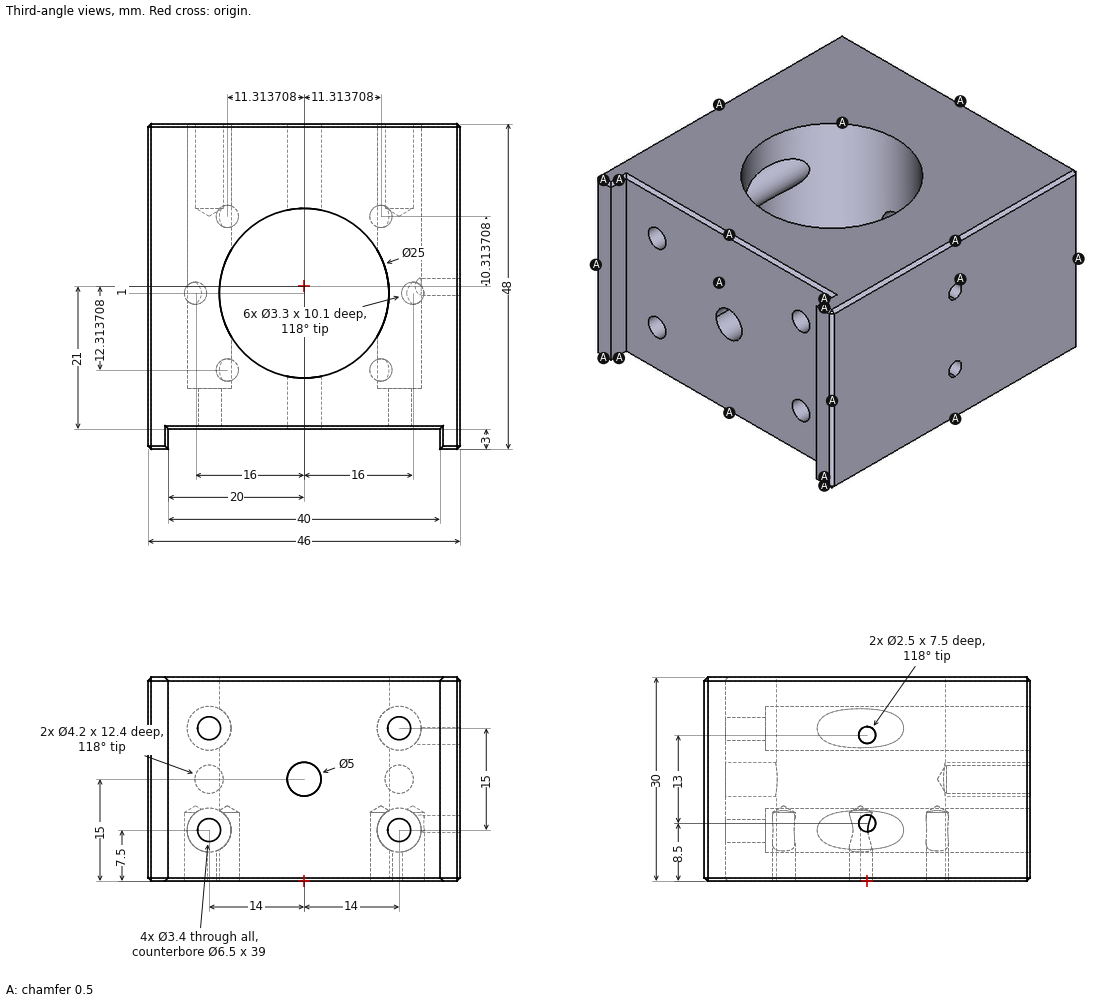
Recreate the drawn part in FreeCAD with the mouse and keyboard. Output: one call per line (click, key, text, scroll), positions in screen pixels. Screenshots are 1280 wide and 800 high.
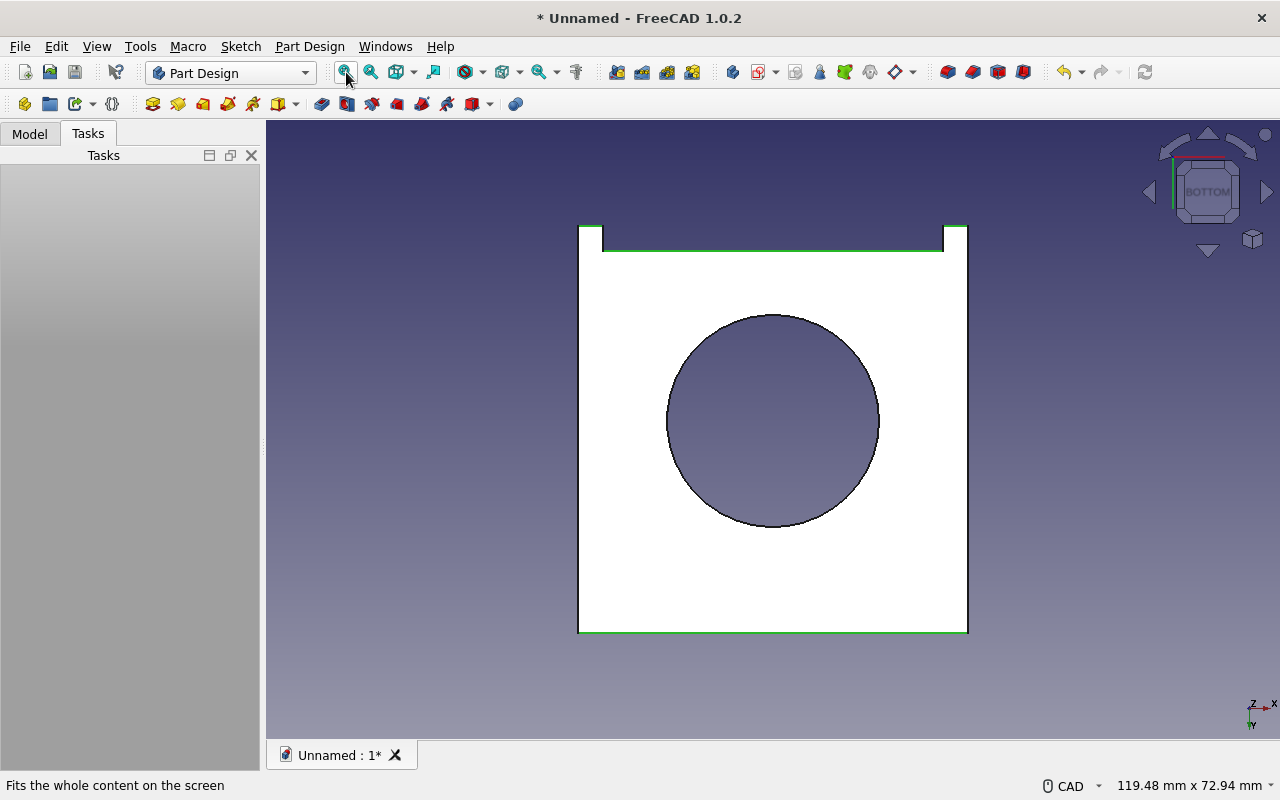
click(603, 238, ctrl)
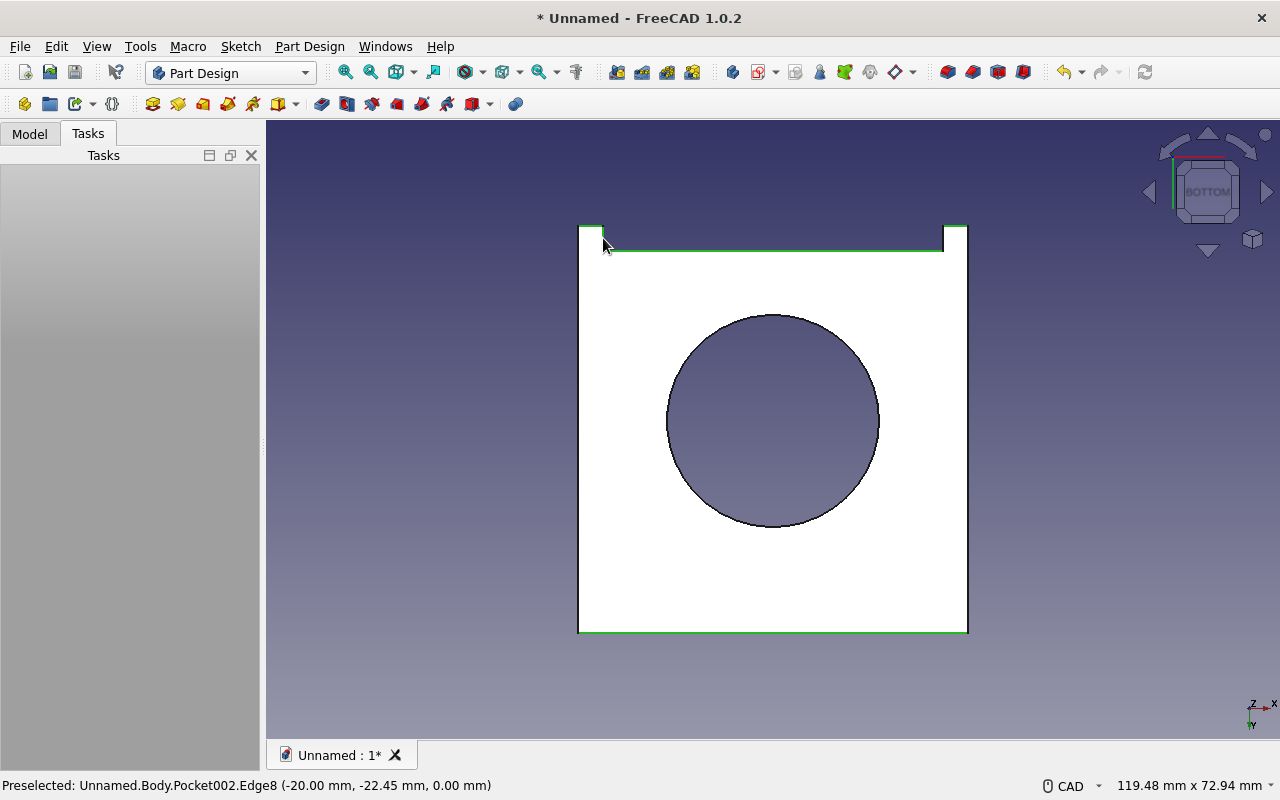
click(943, 238, ctrl)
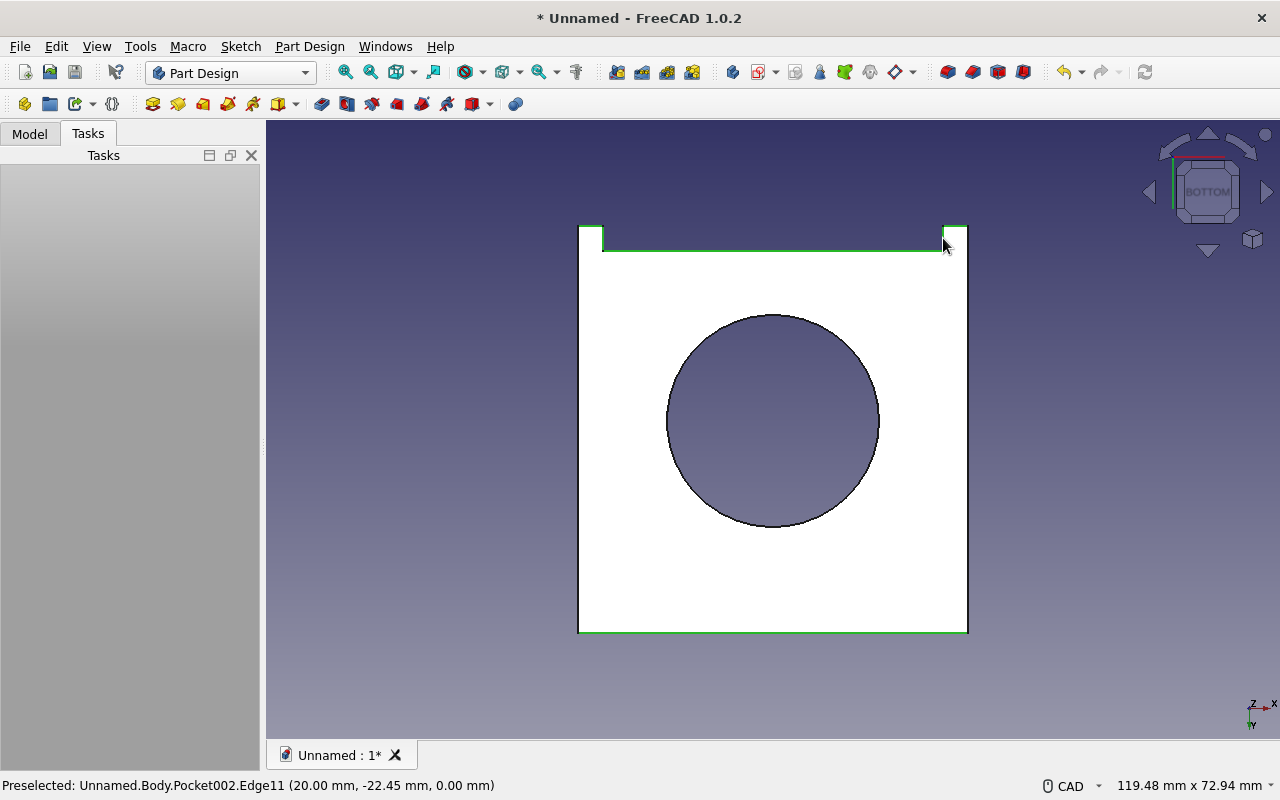
key(4)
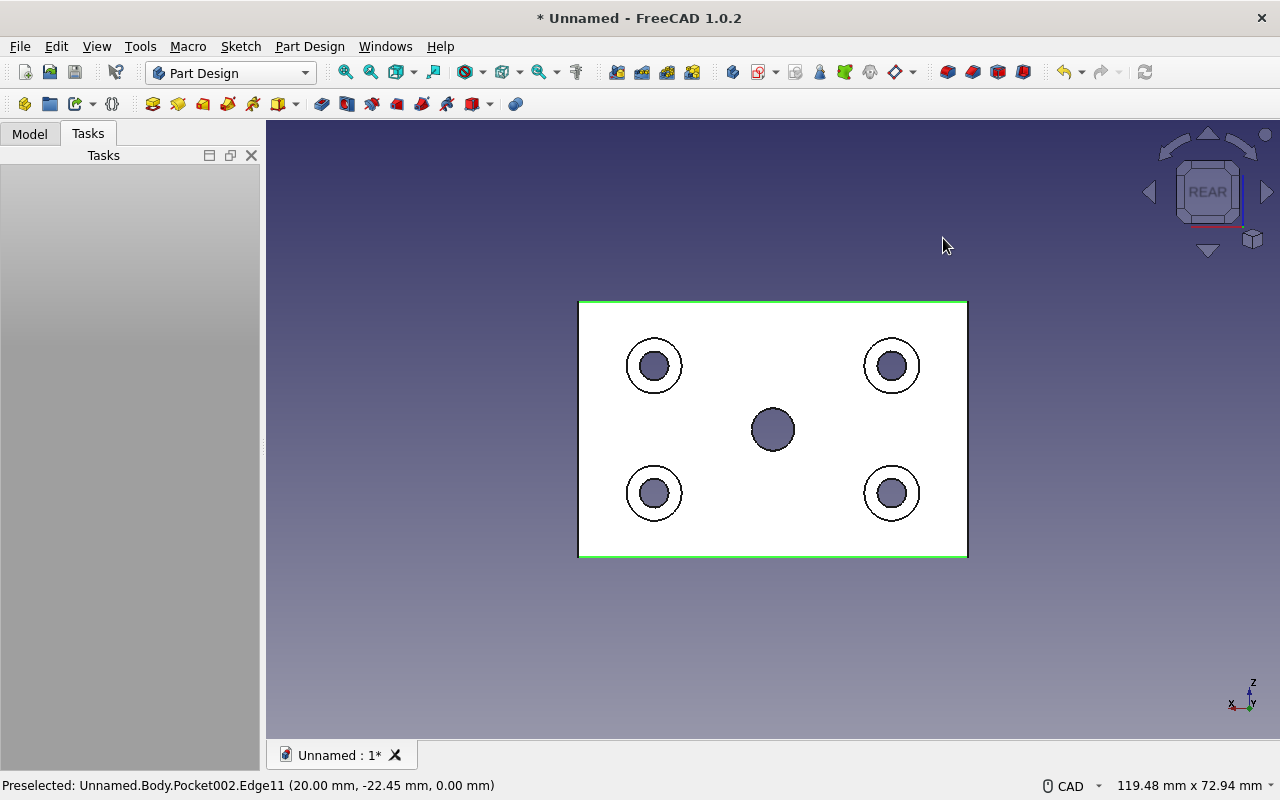
click(346, 72)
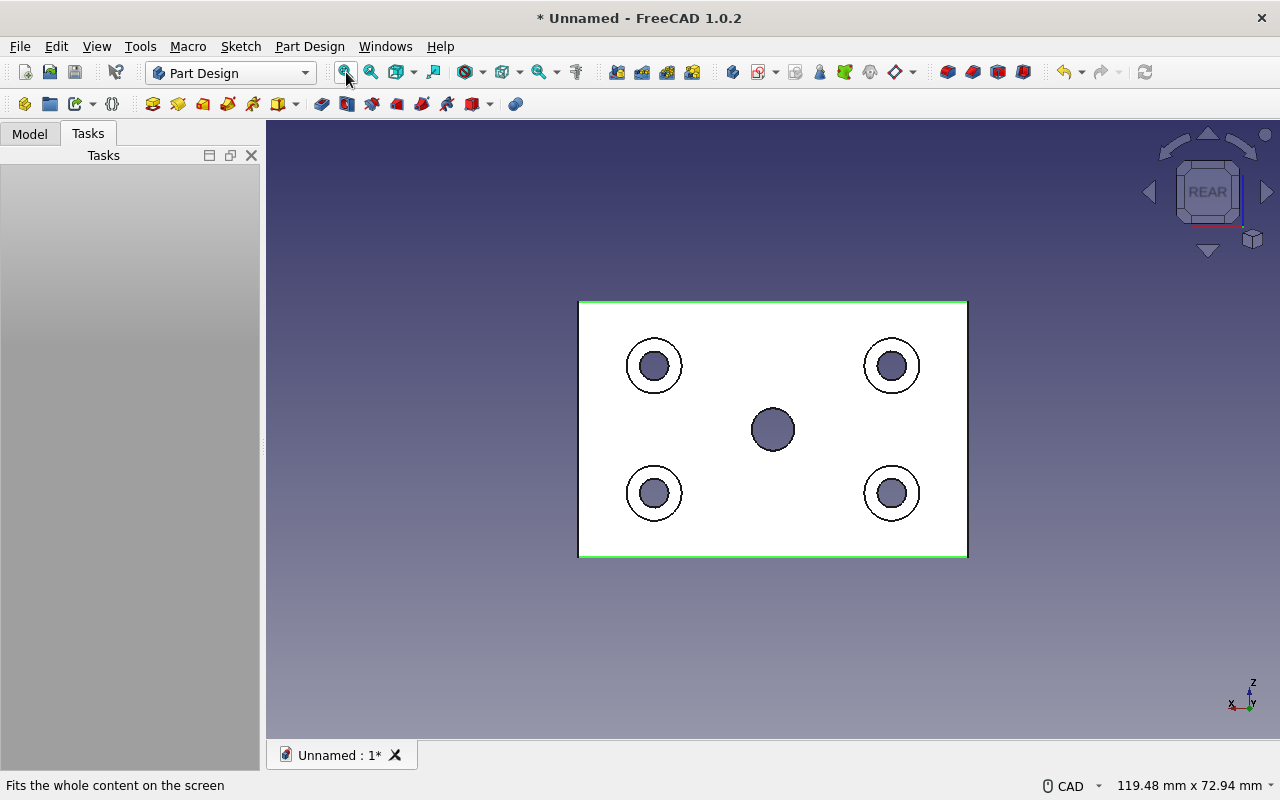
key(6)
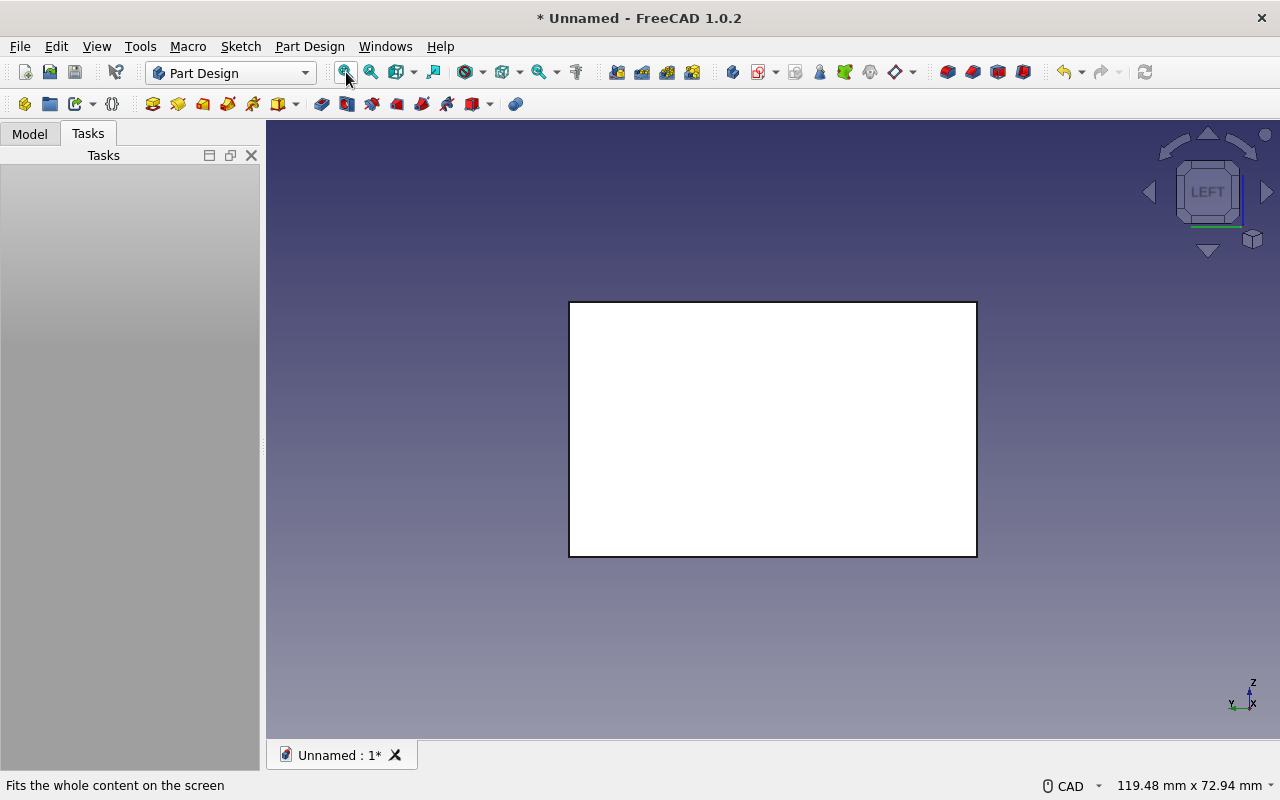
click(346, 72)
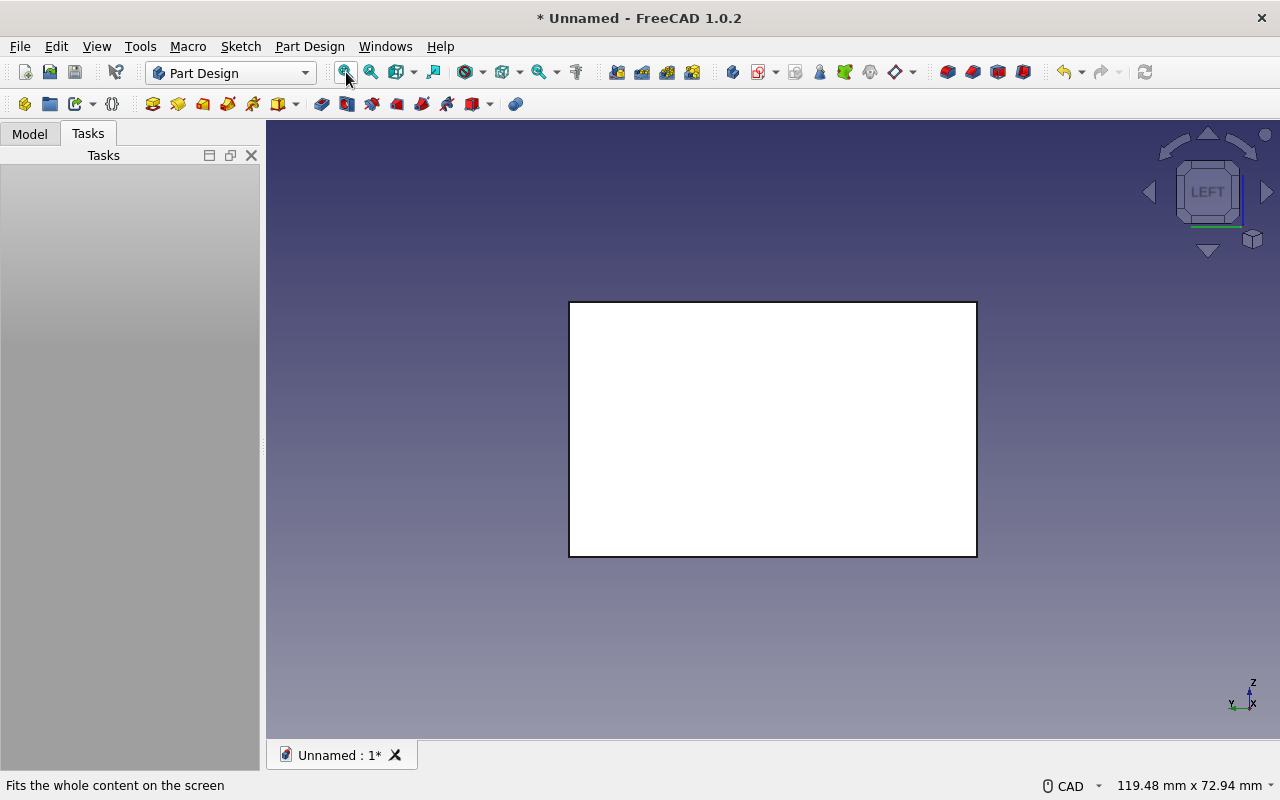
click(715, 428, ctrl)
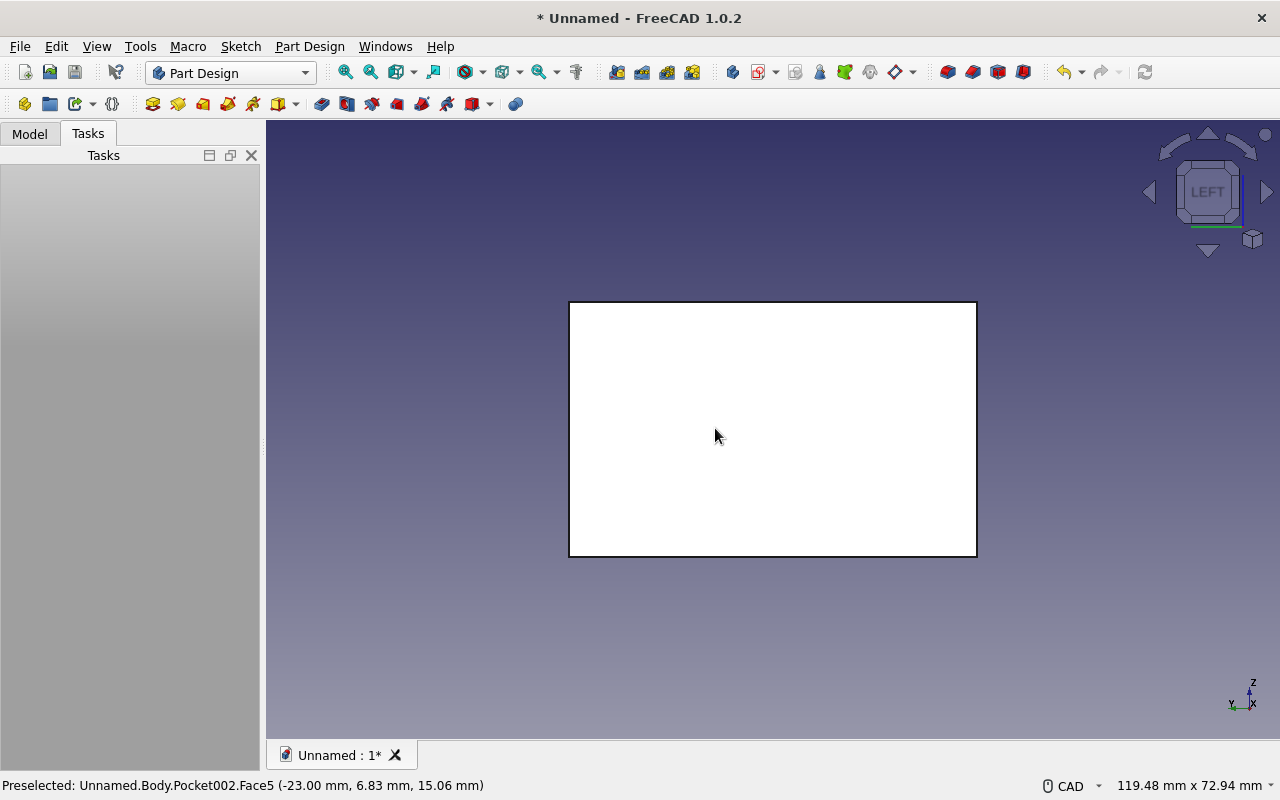
click(973, 72)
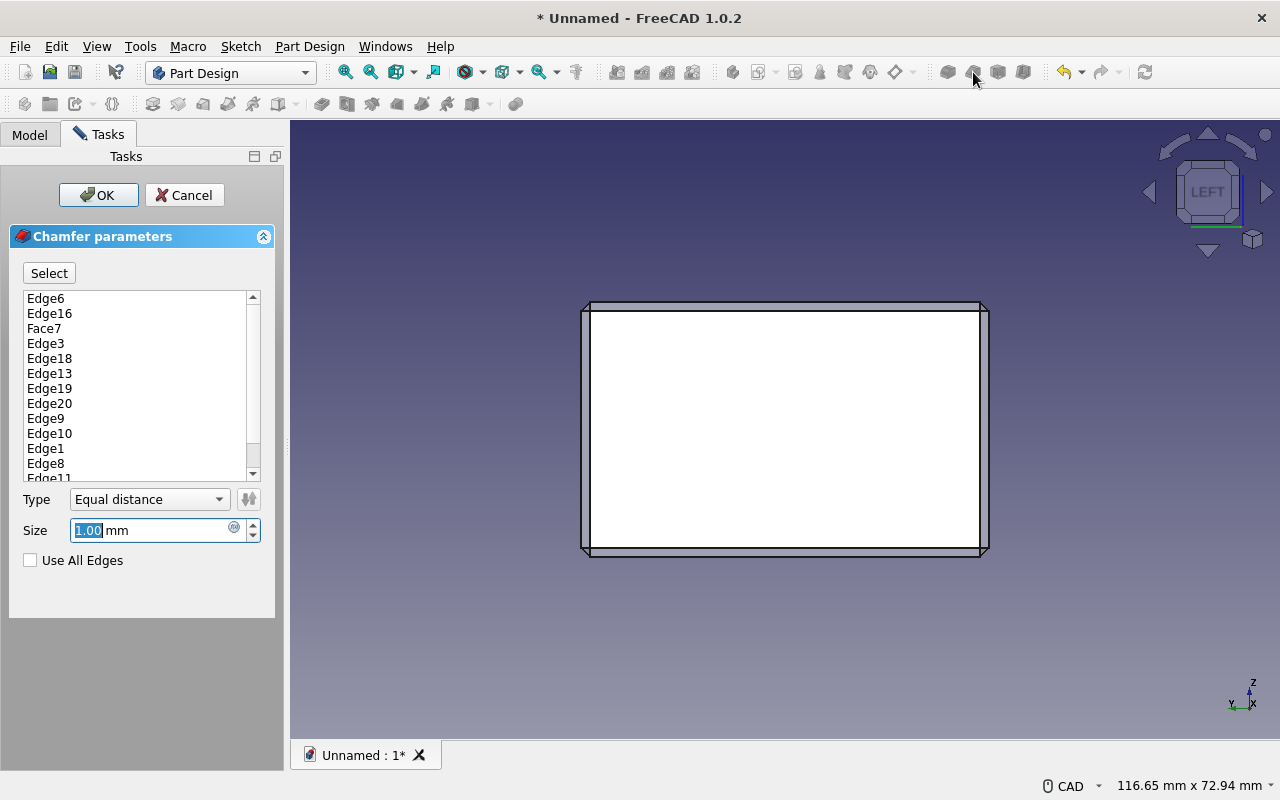
text(0.5)
key(Tab)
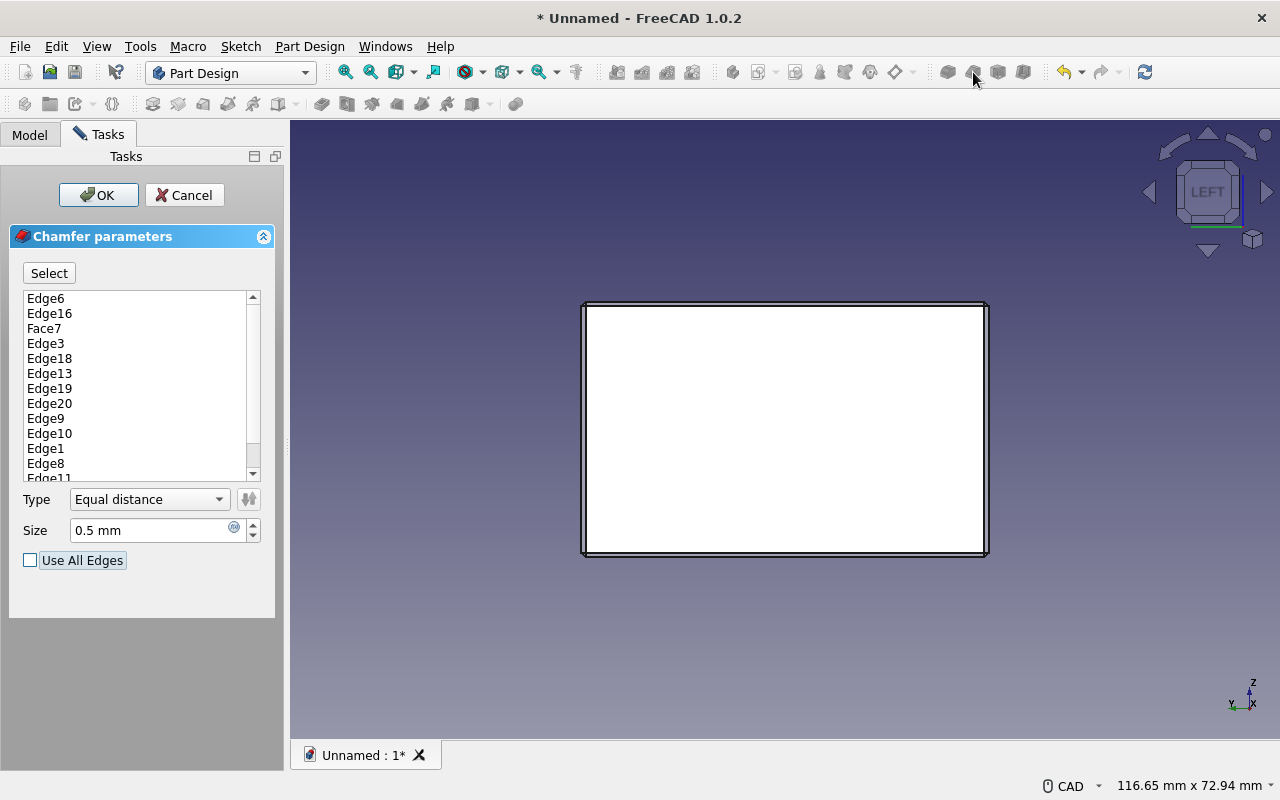
click(99, 195)